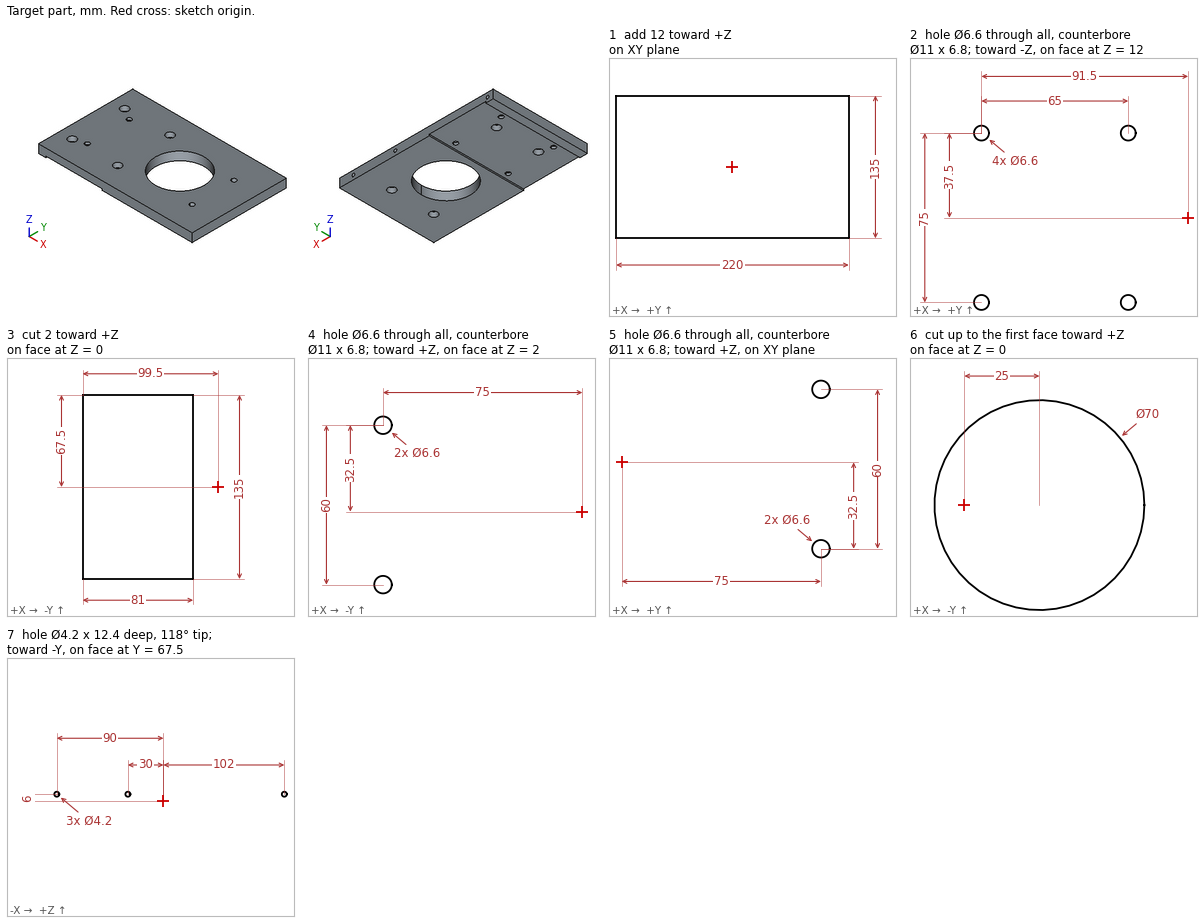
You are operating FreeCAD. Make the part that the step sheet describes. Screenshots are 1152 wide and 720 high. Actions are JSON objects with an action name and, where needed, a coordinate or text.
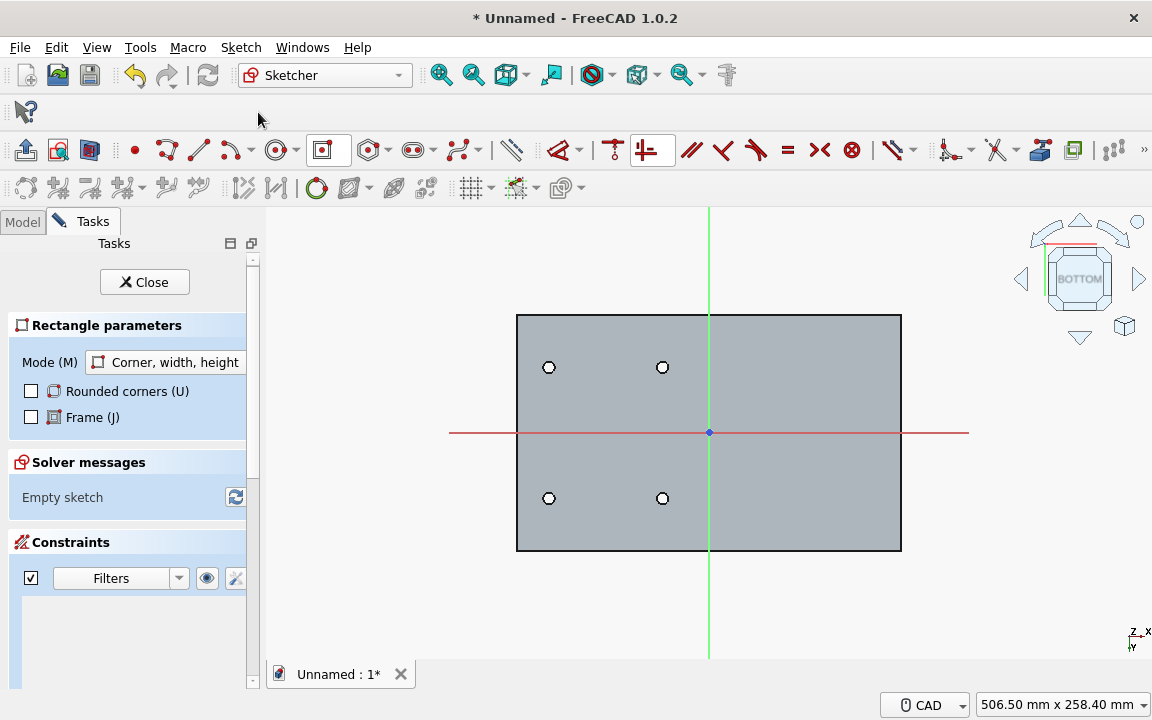
{"action": "left_click", "coordinate": [535, 315]}
{"action": "mouse_move", "coordinate": [677, 551]}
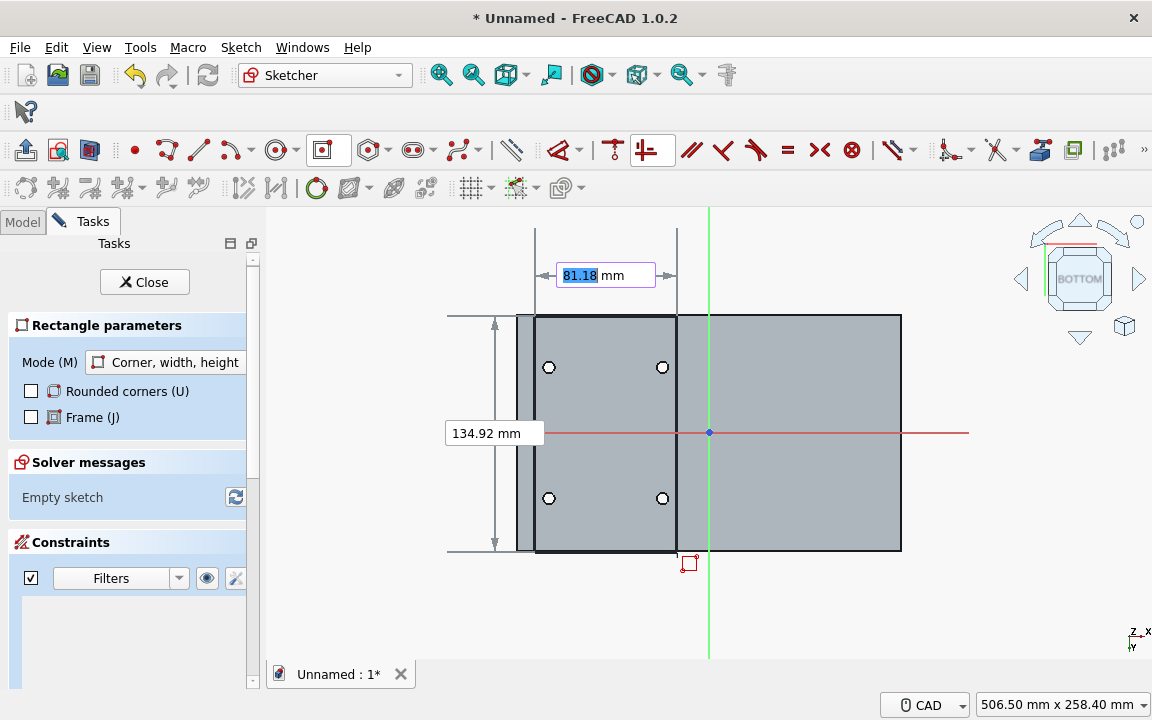
{"action": "type", "text": "81"}
{"action": "key", "text": "Tab"}
{"action": "type", "text": "135"}
{"action": "key", "text": "Return"}
{"action": "key", "text": "Escape"}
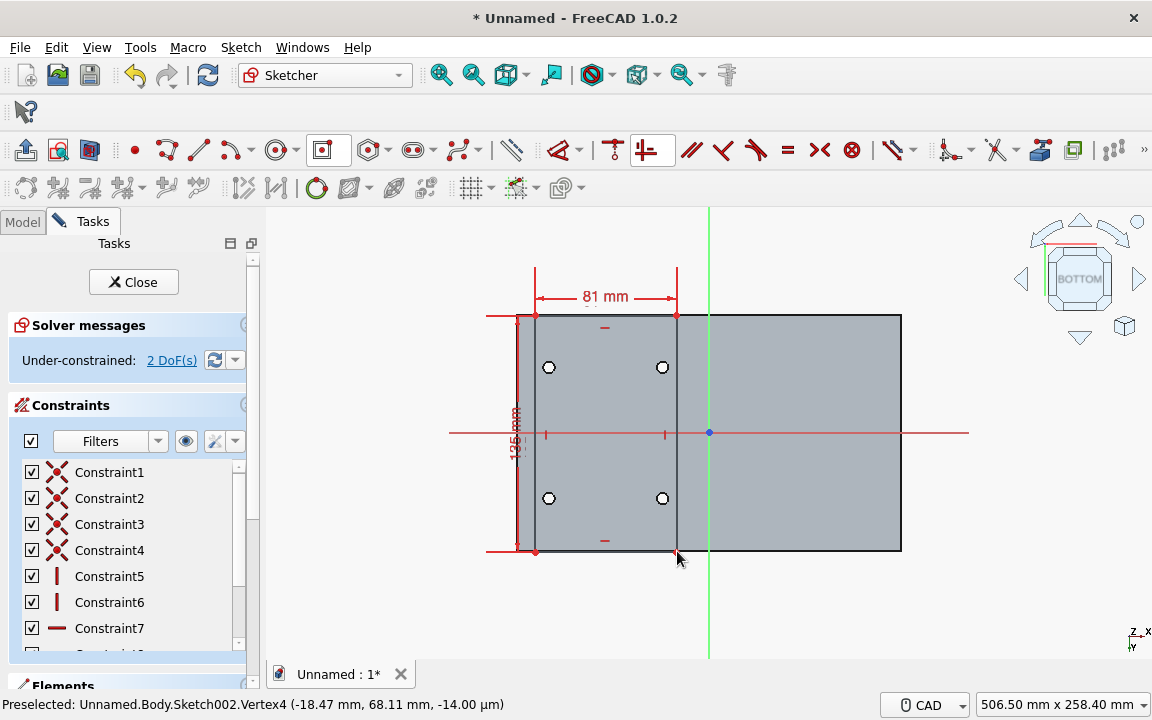
{"action": "left_click", "coordinate": [558, 150]}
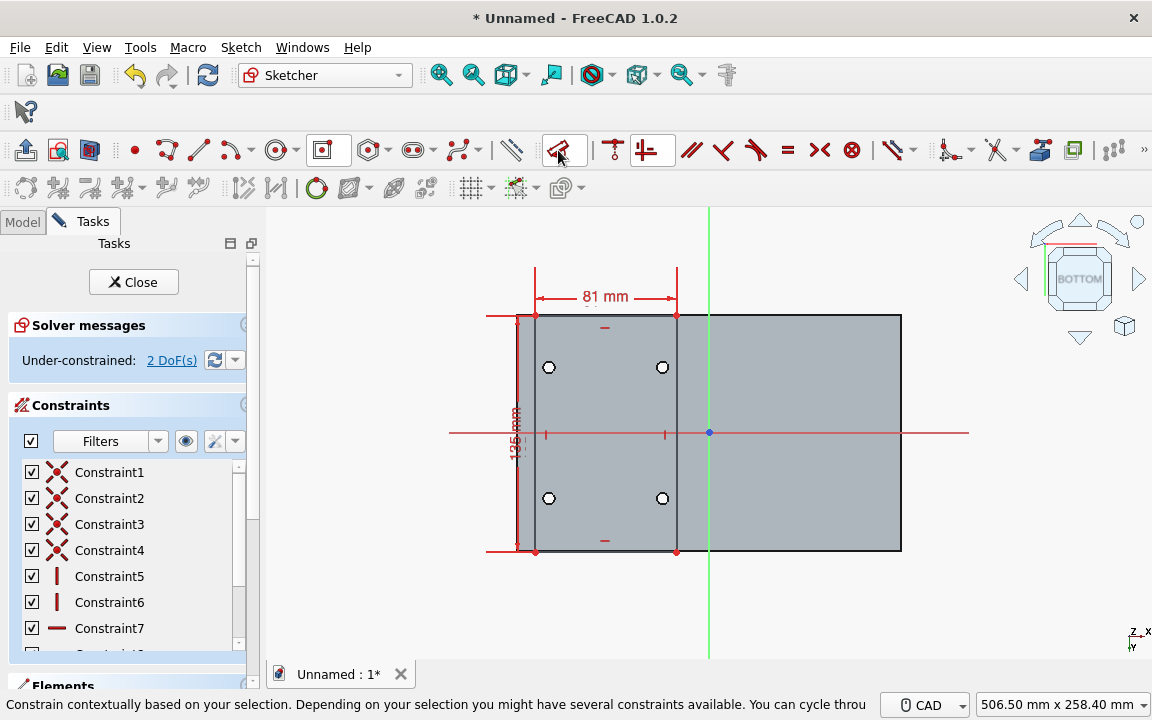
{"action": "left_click", "coordinate": [535, 316]}
{"action": "left_click", "coordinate": [622, 282]}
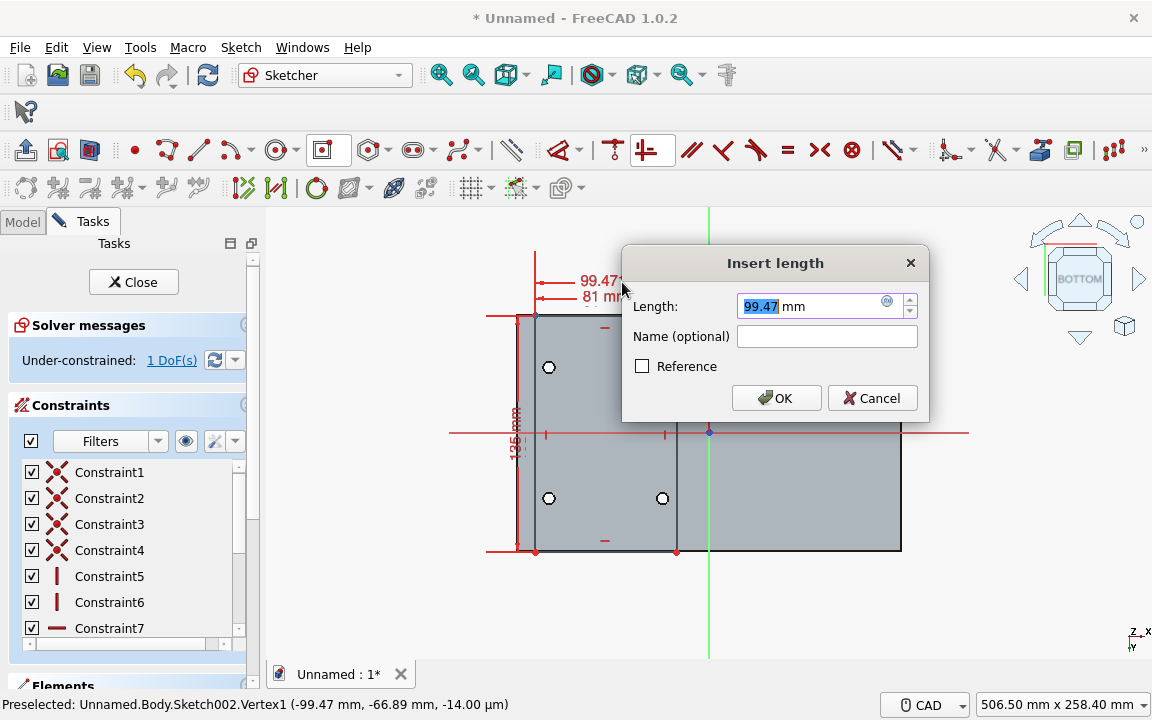
{"action": "type", "text": "99.5"}
{"action": "key", "text": "Return"}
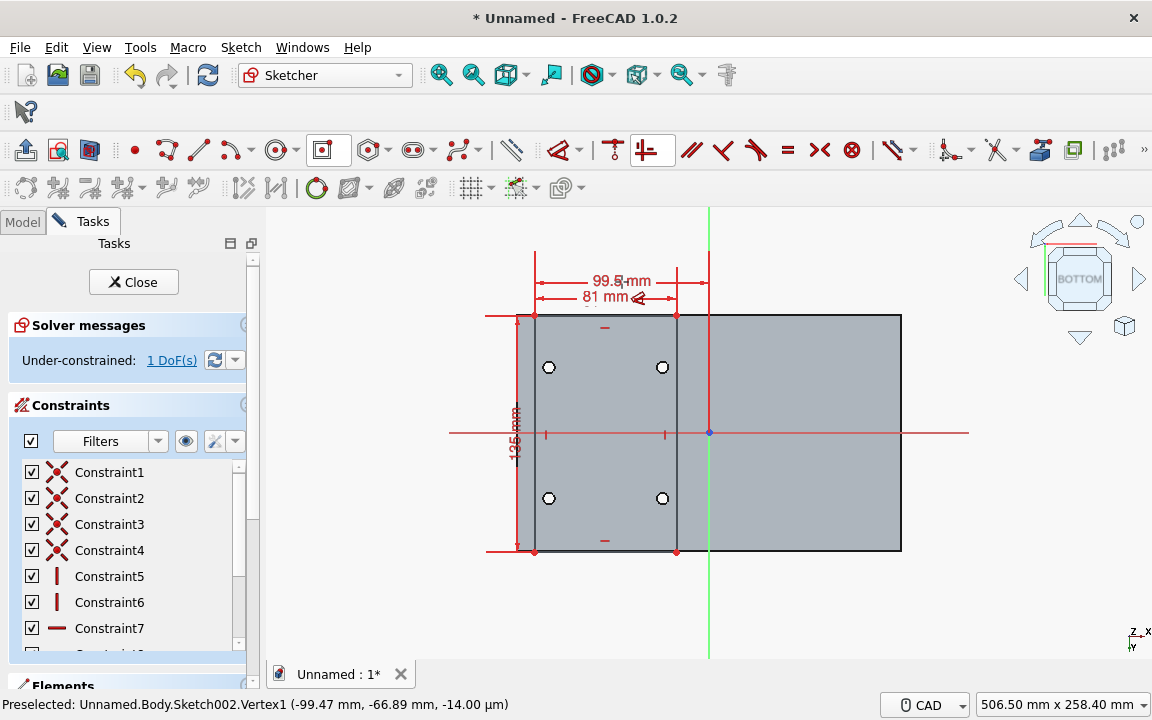
{"action": "left_click", "coordinate": [535, 316]}
{"action": "left_click", "coordinate": [743, 375]}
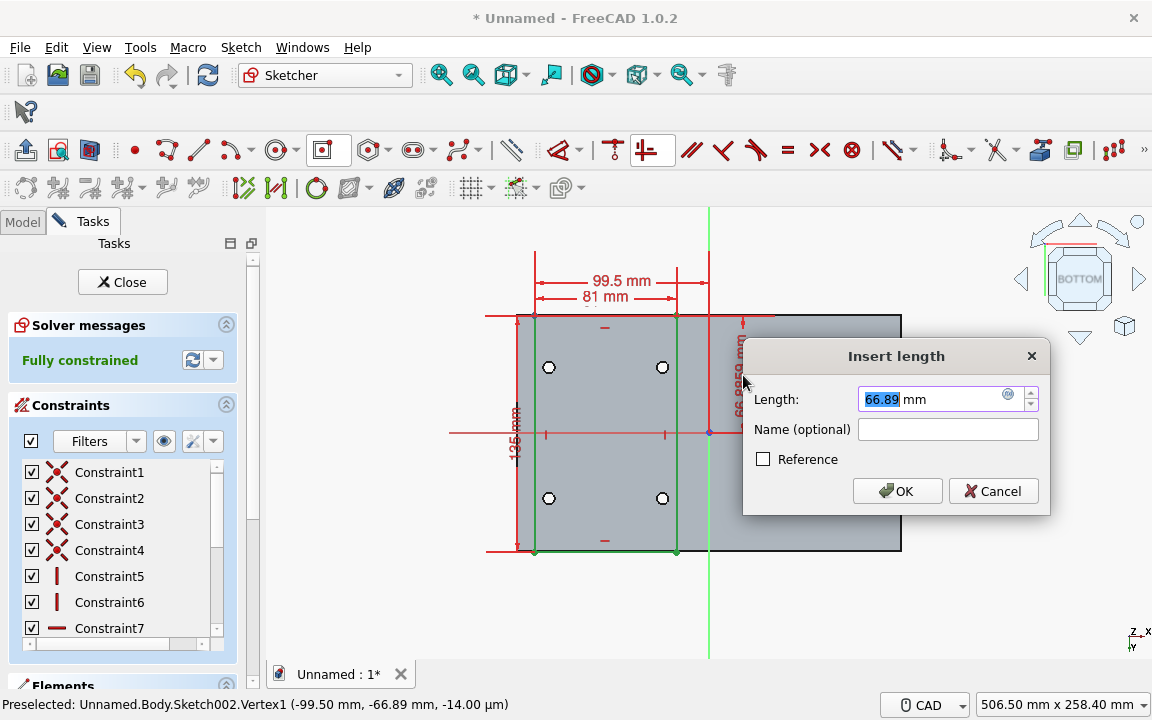
{"action": "type", "text": "67.5"}
{"action": "key", "text": "Return"}
{"action": "key", "text": "Escape"}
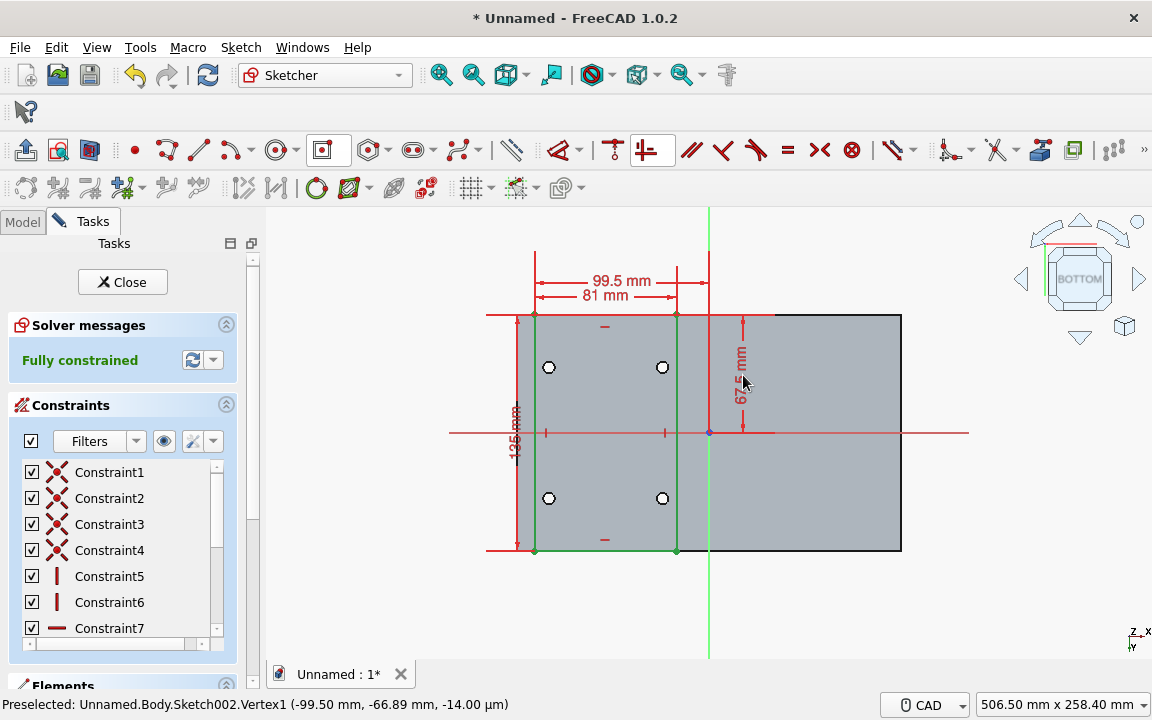
{"action": "left_click", "coordinate": [123, 282]}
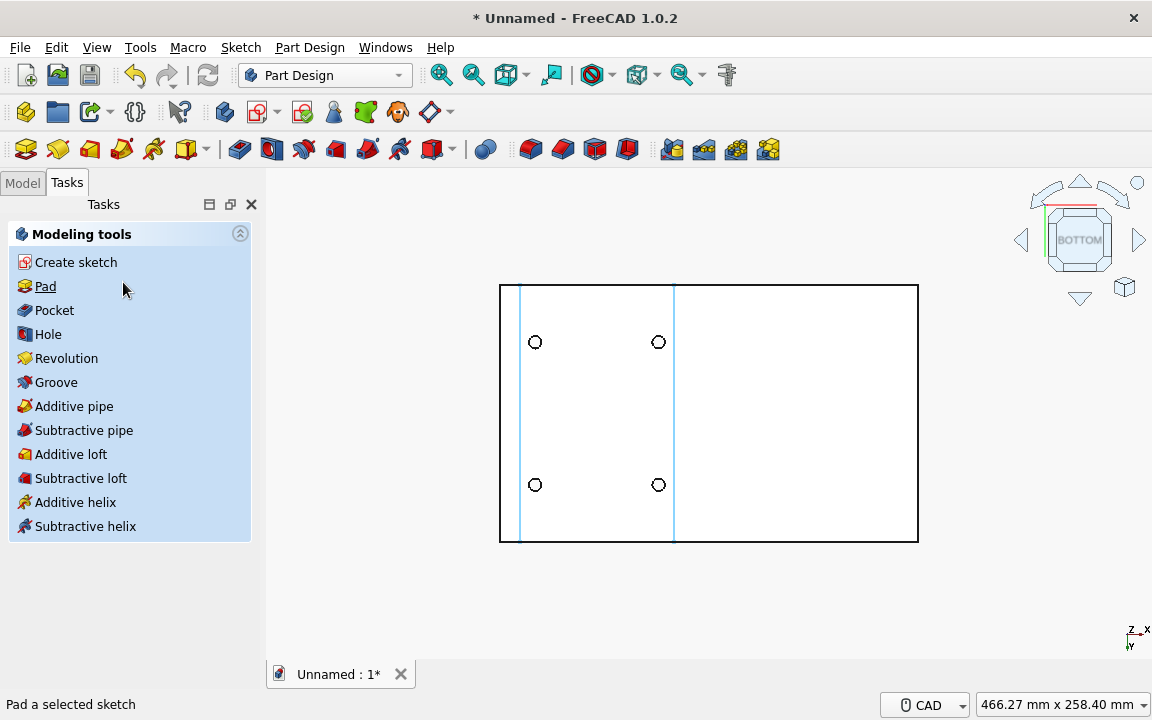
{"action": "left_click", "coordinate": [240, 150]}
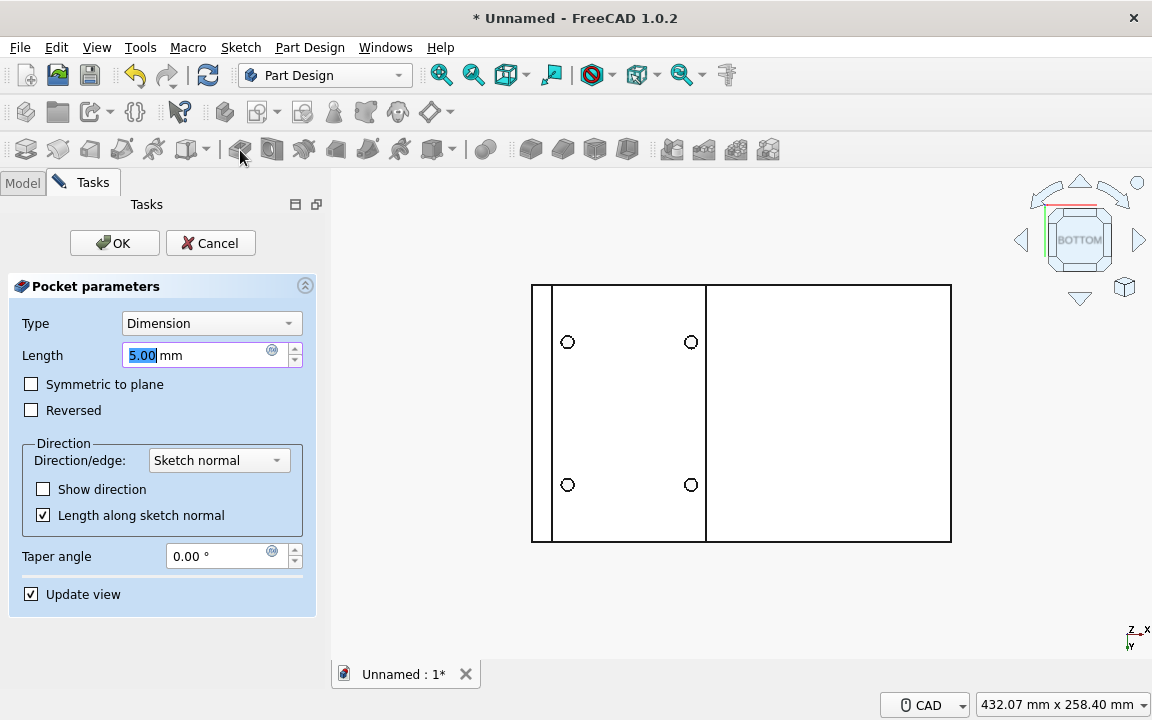
{"action": "type", "text": "2"}
{"action": "key", "text": "Tab"}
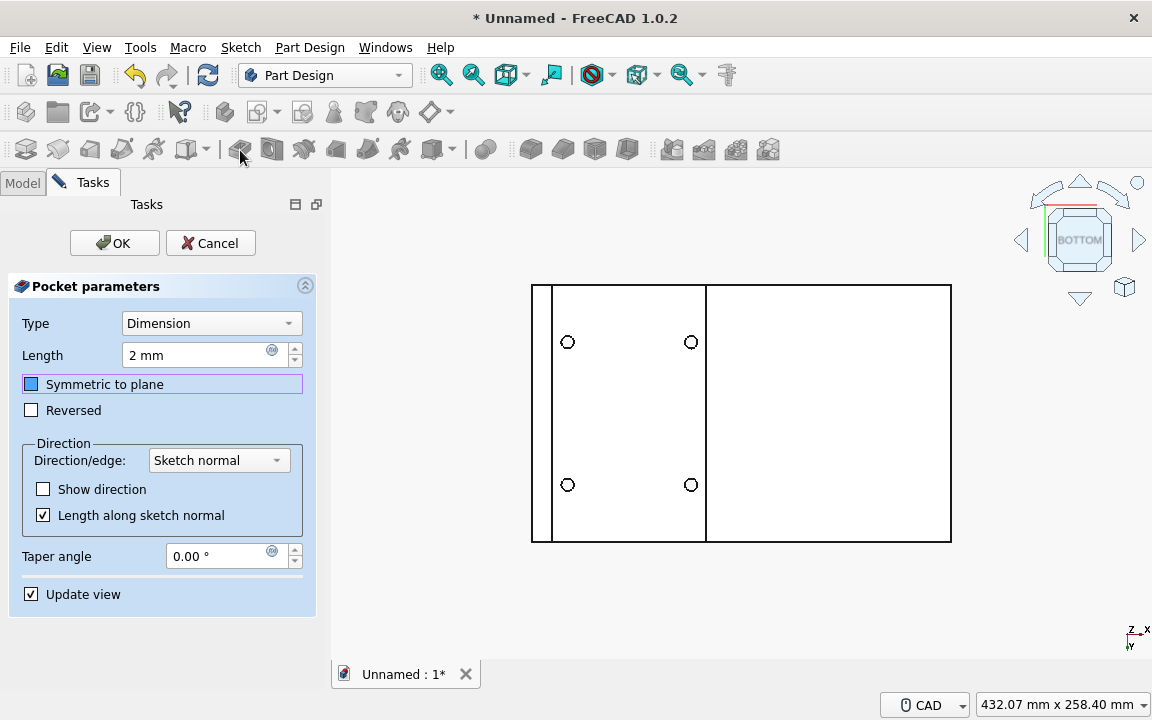
{"action": "left_click", "coordinate": [115, 243]}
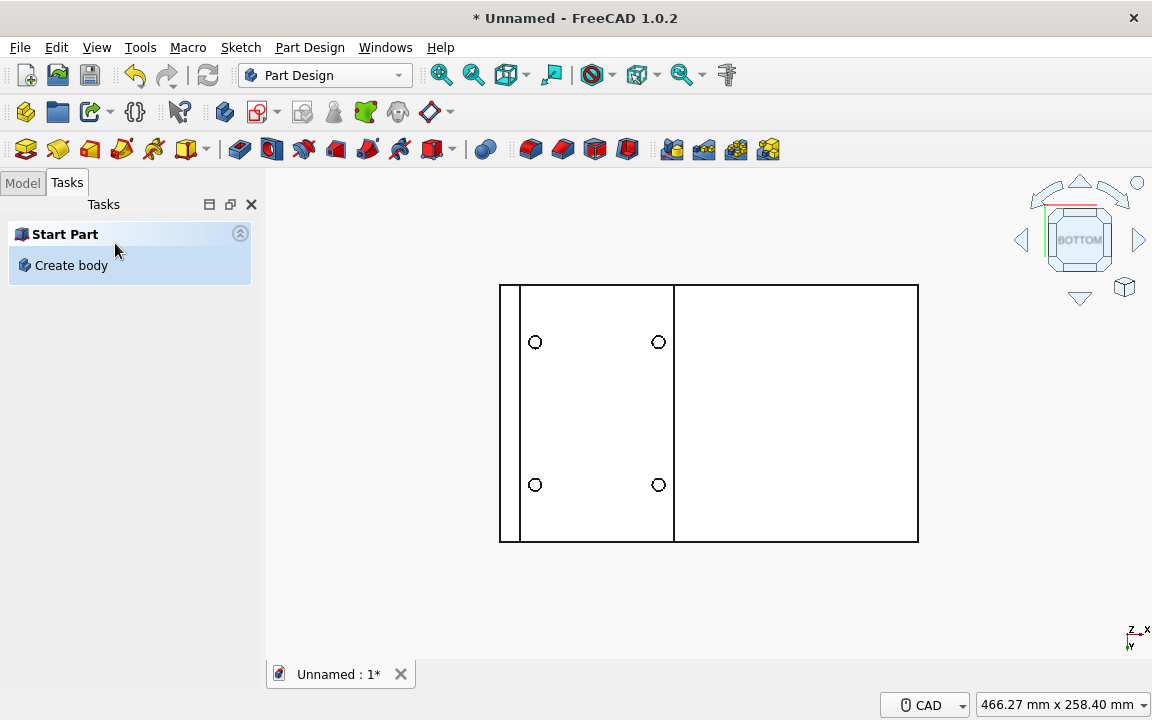
{"action": "left_click", "coordinate": [597, 413]}